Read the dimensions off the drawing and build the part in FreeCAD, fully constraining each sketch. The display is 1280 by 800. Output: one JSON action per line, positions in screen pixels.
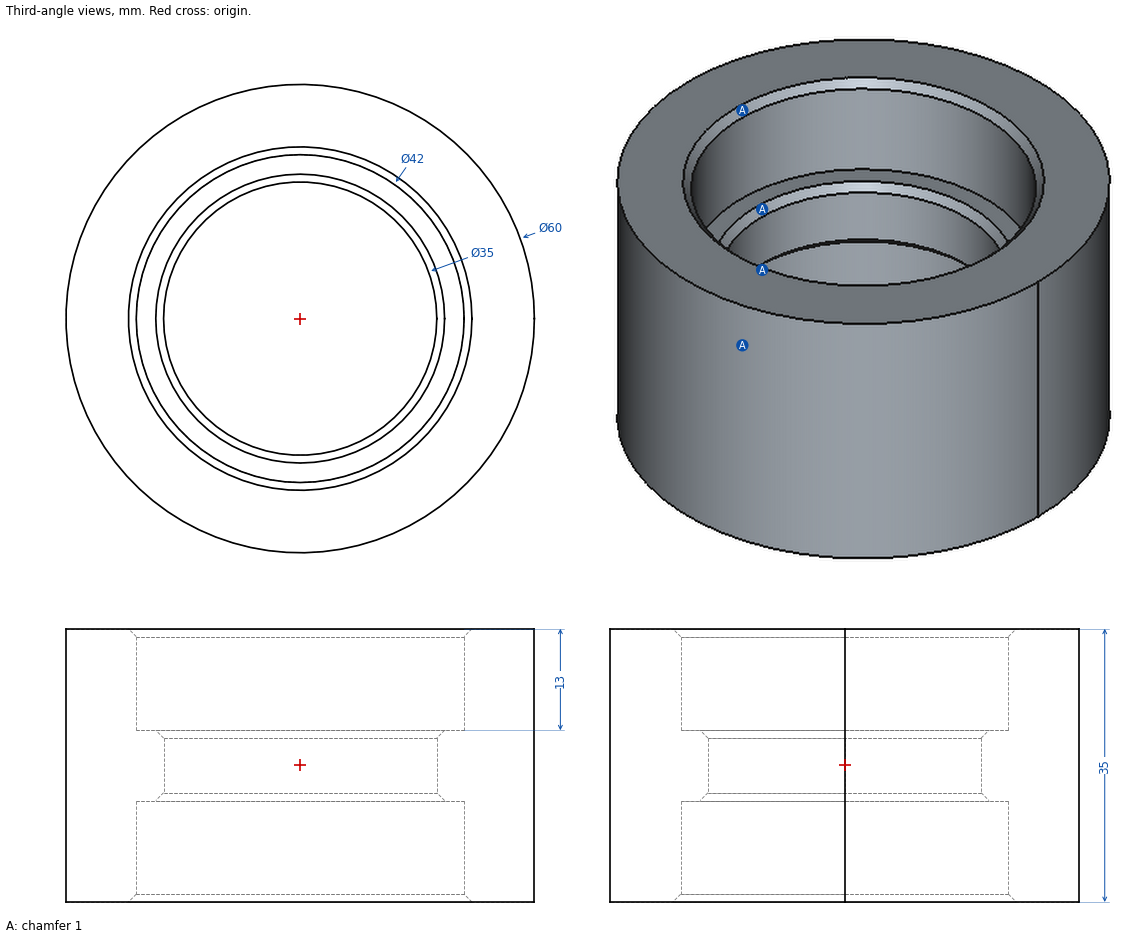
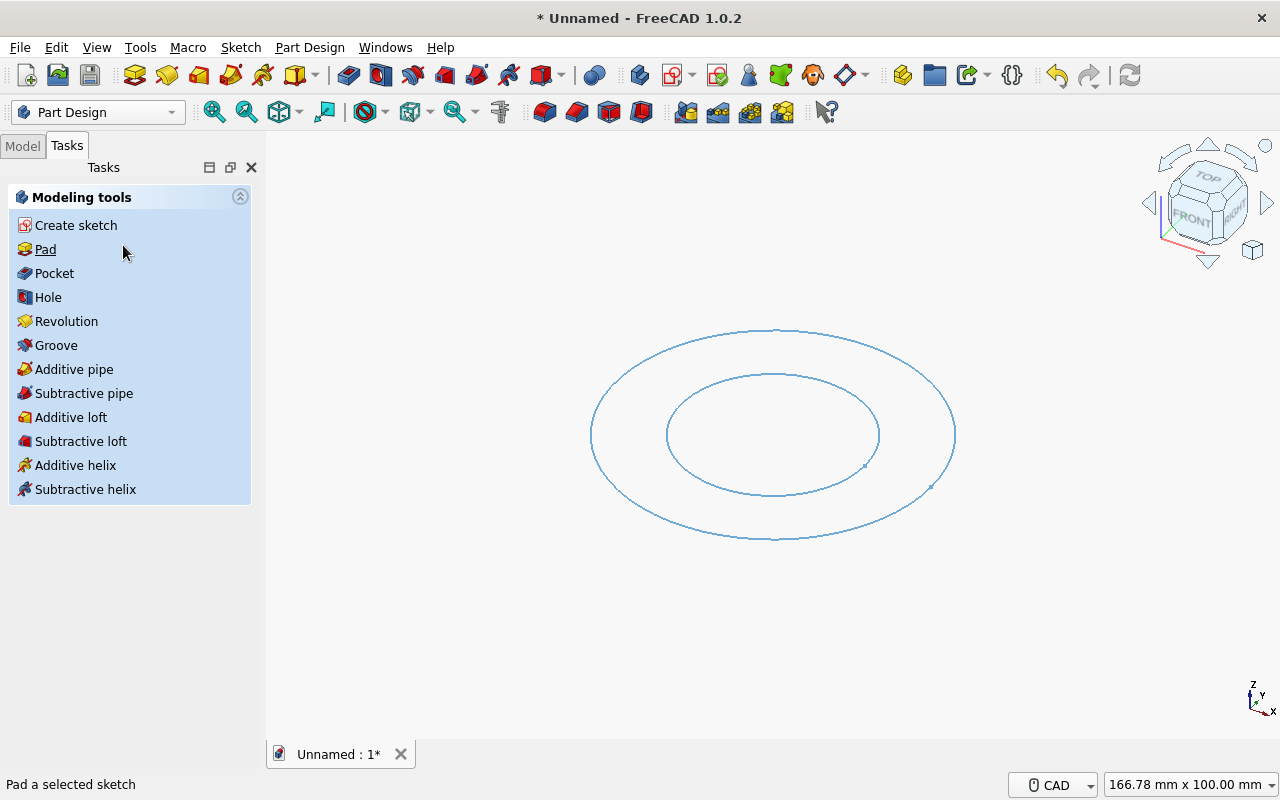
{"action": "left_click", "coordinate": [136, 76]}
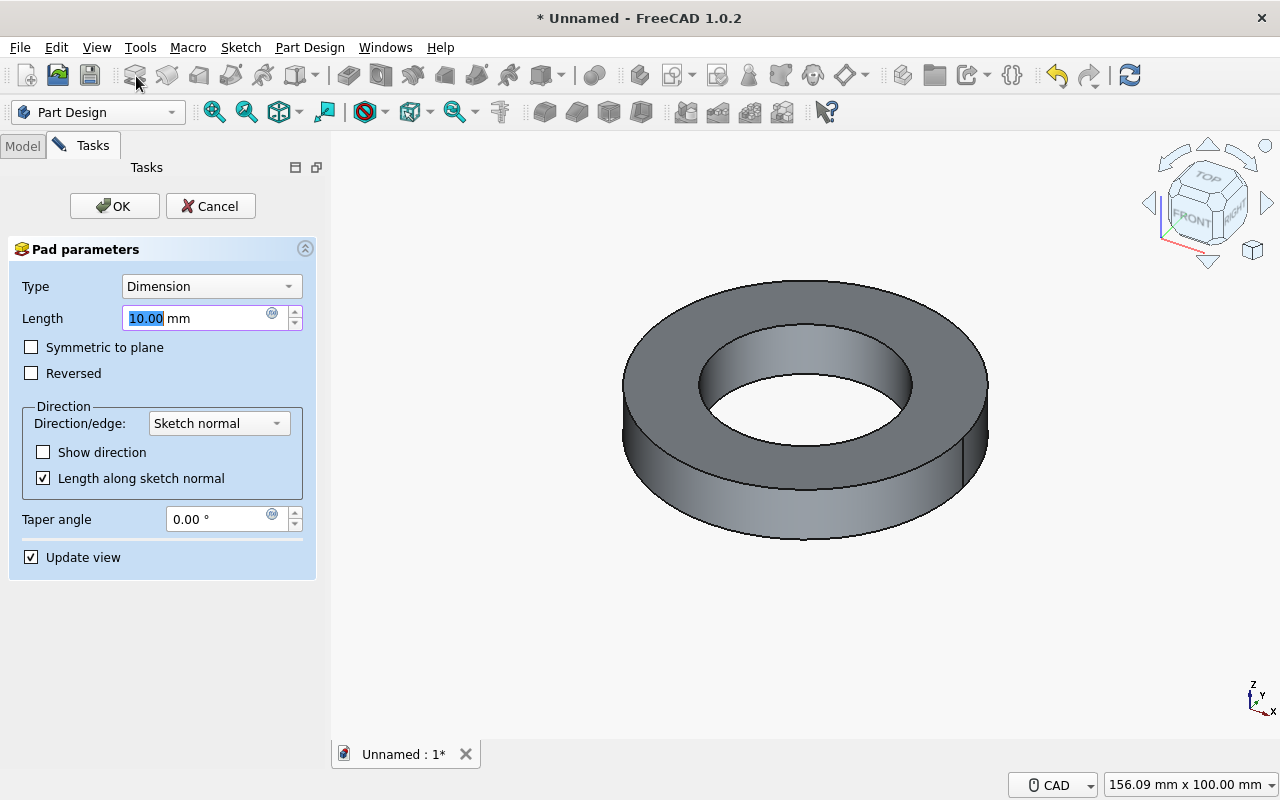
{"action": "type", "text": "35"}
{"action": "key", "text": "Tab"}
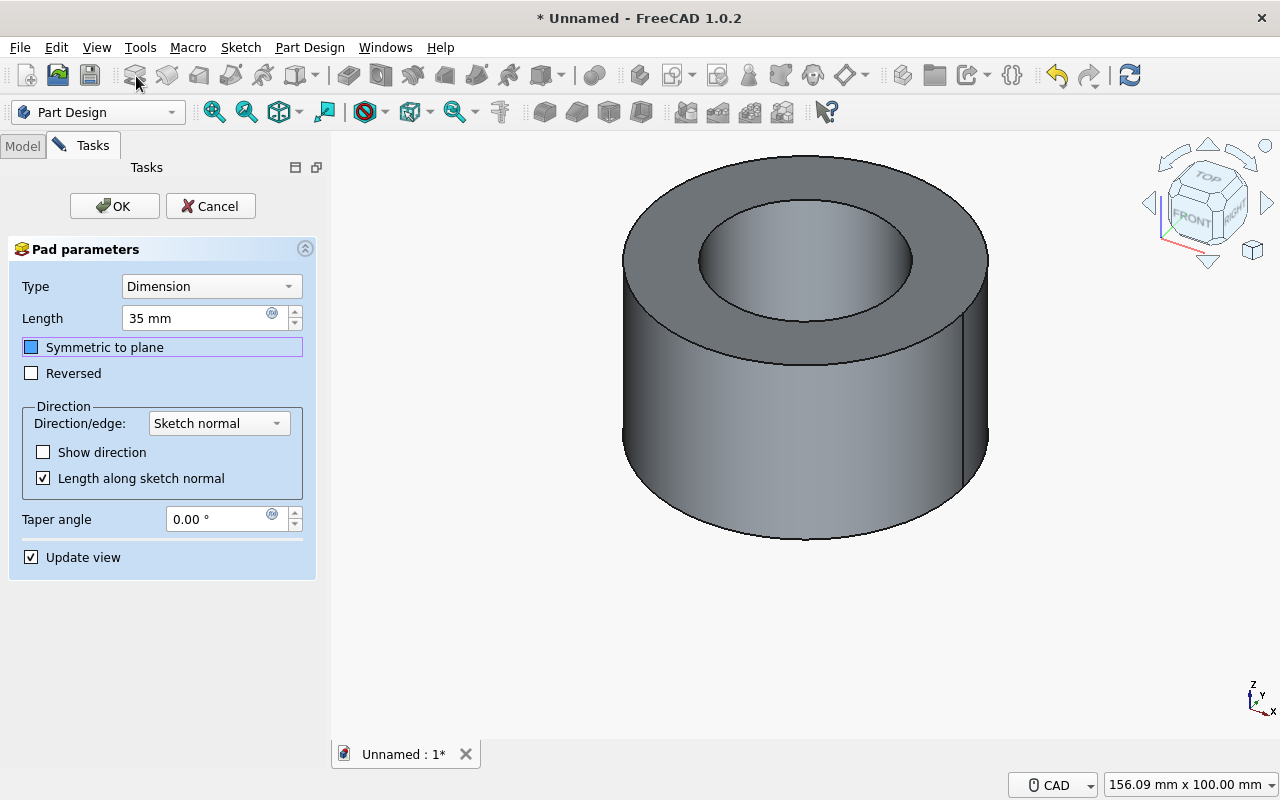
{"action": "left_click", "coordinate": [30, 347]}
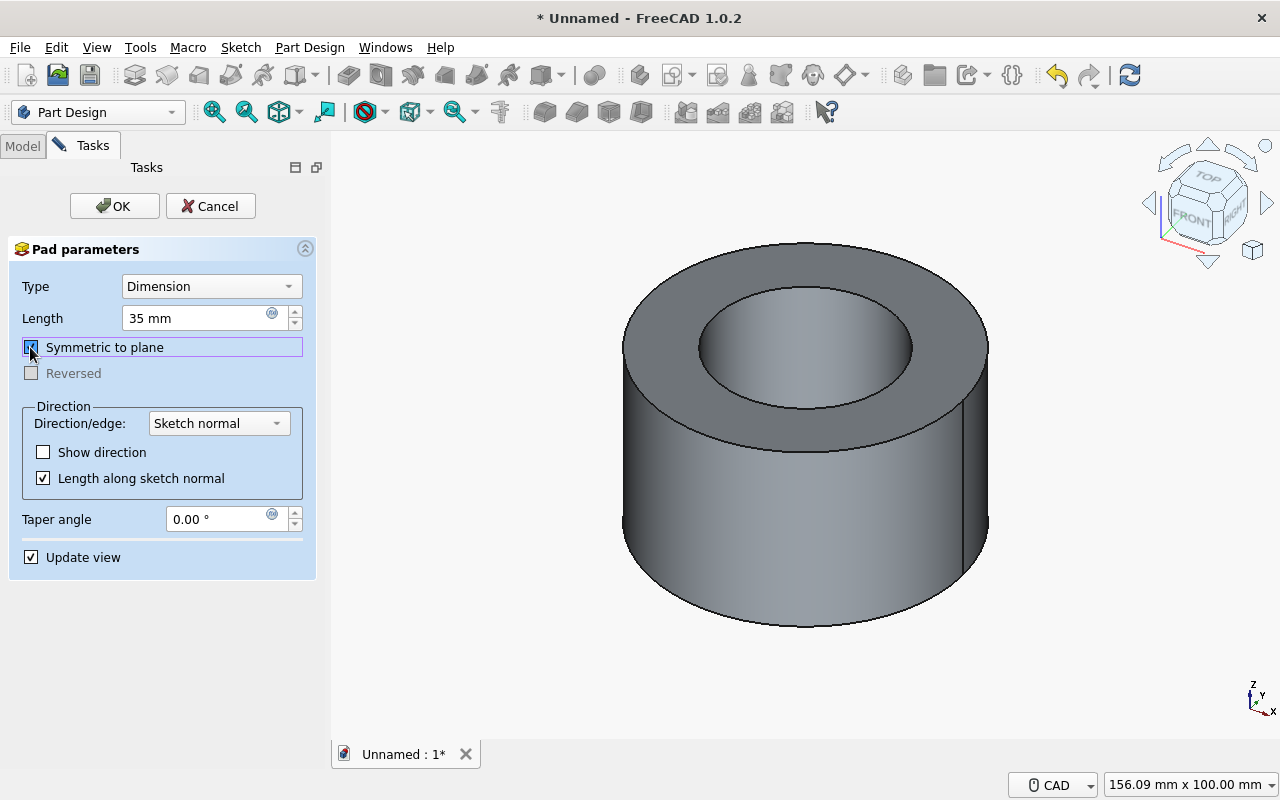
{"action": "left_click", "coordinate": [115, 206]}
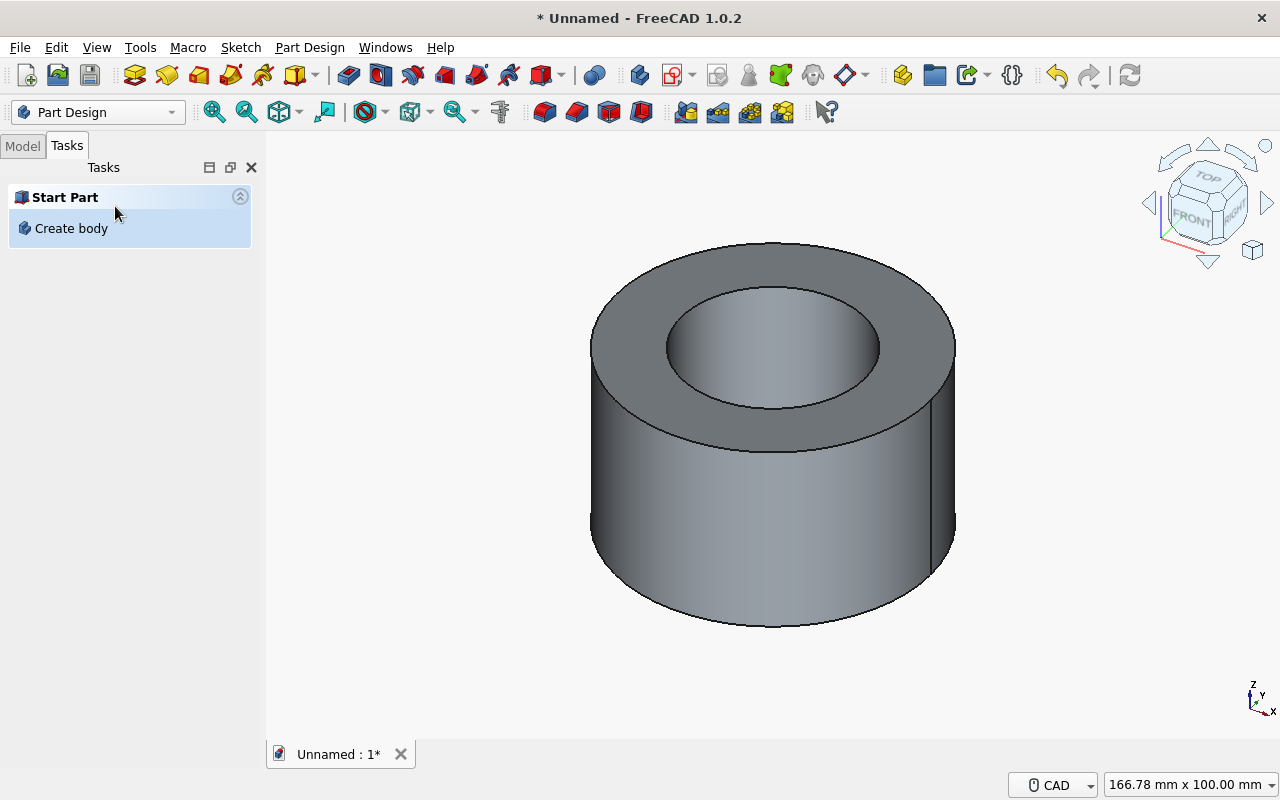
{"action": "left_click", "coordinate": [631, 369]}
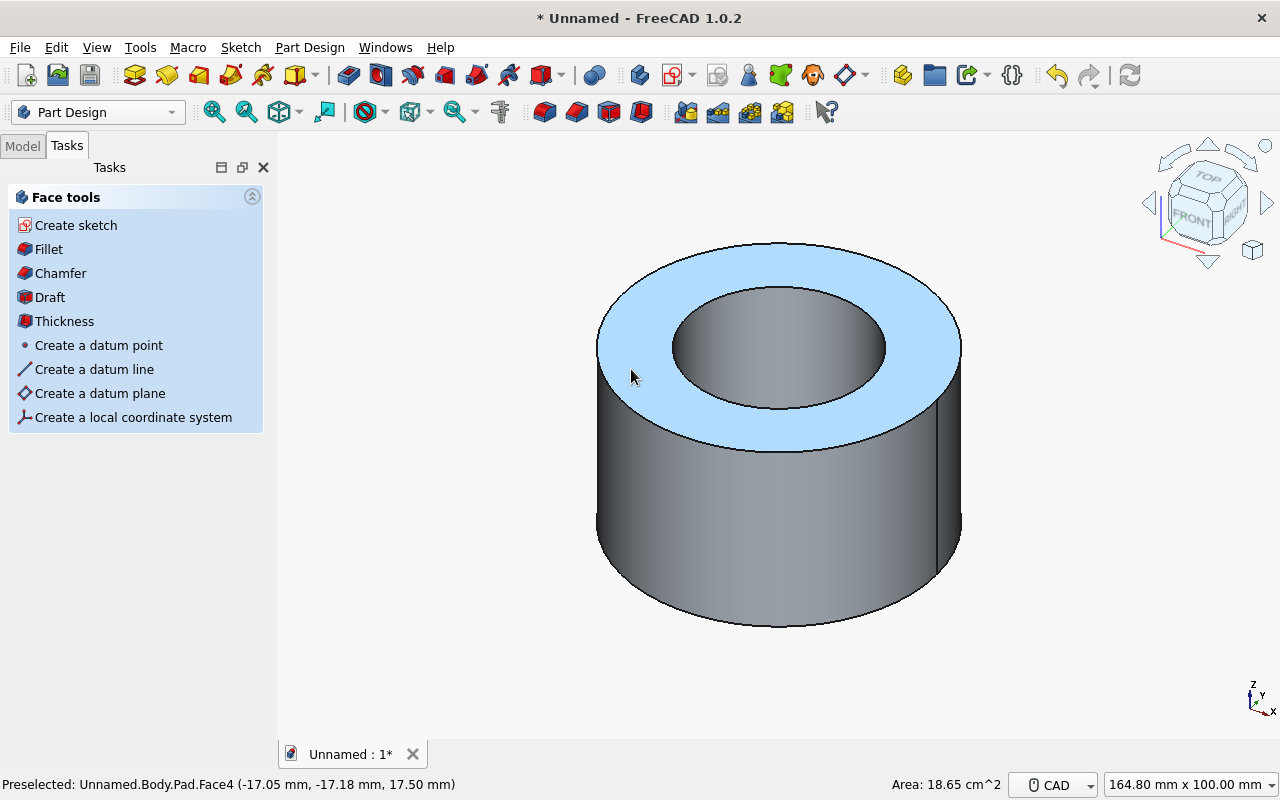
{"action": "left_click", "coordinate": [672, 76]}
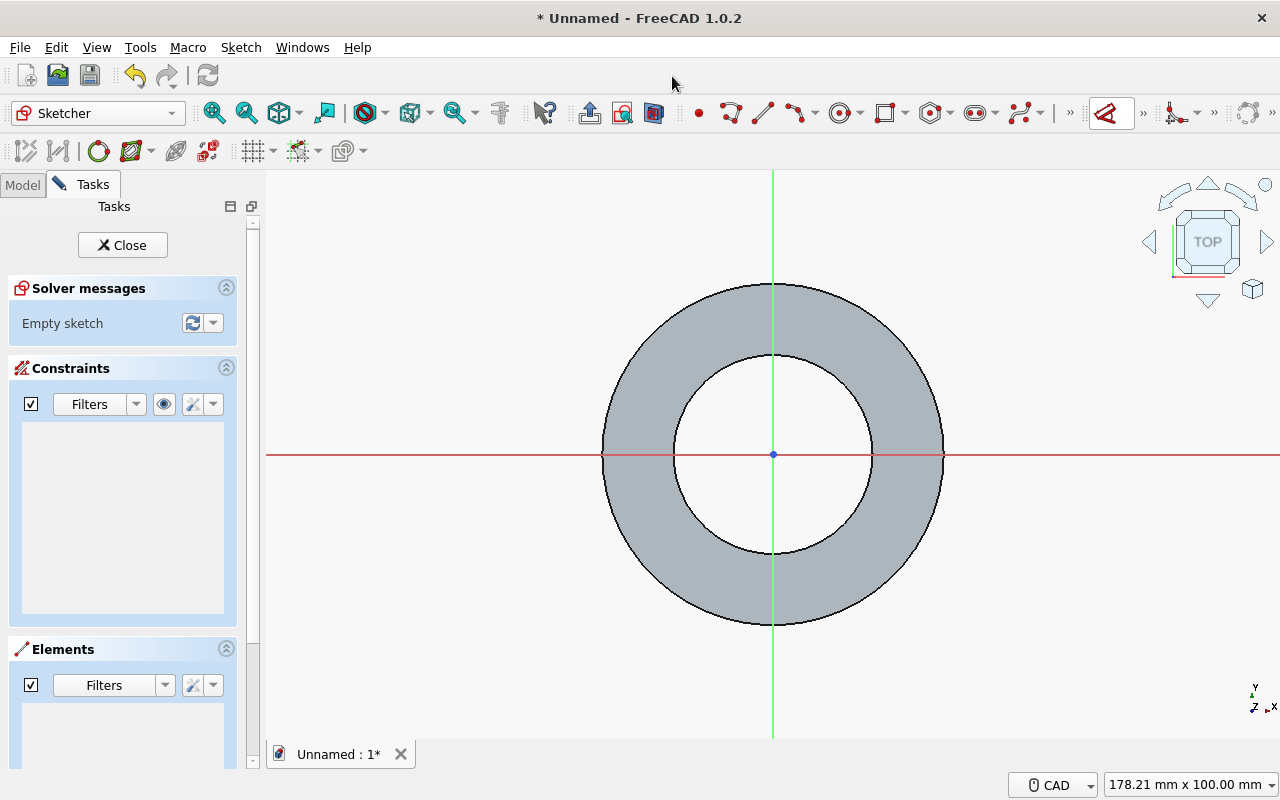
{"action": "scroll", "coordinate": [912, 455], "scroll_direction": "up", "scroll_amount": 2}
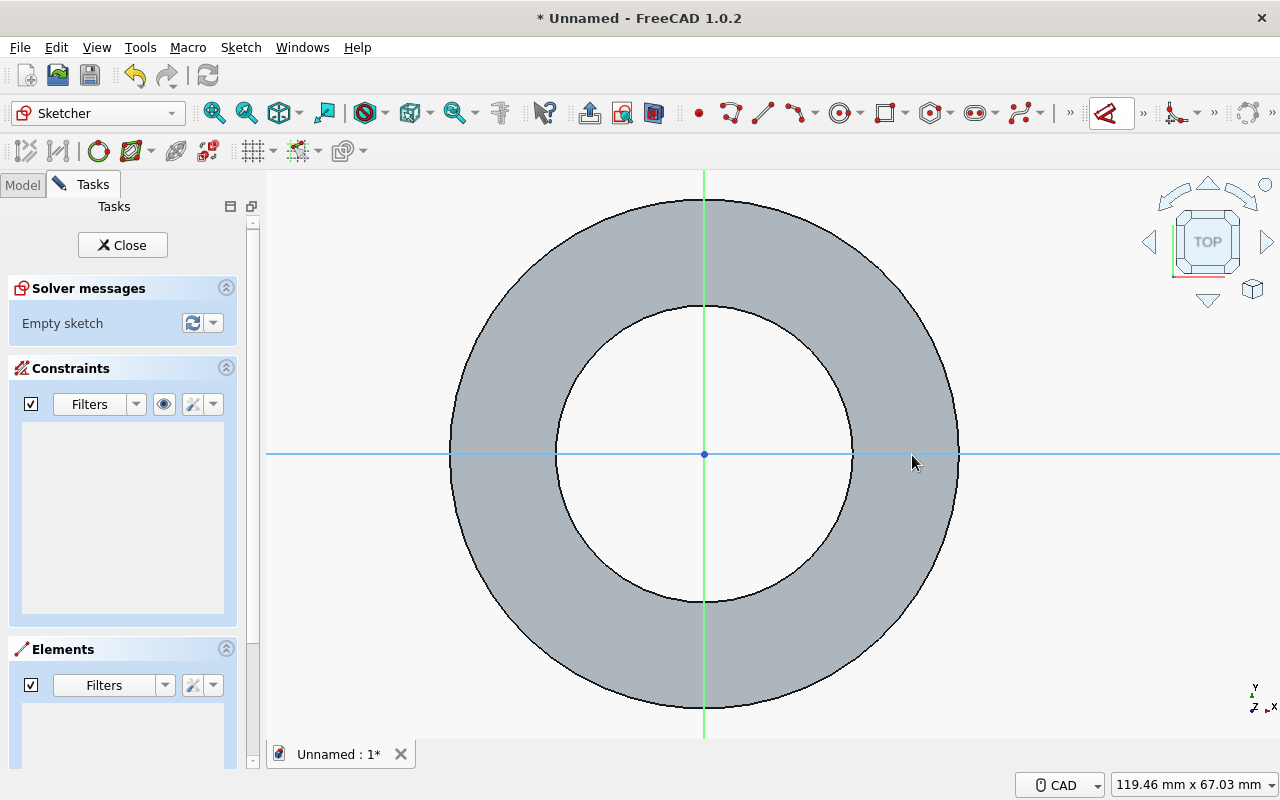
{"action": "left_click", "coordinate": [840, 114]}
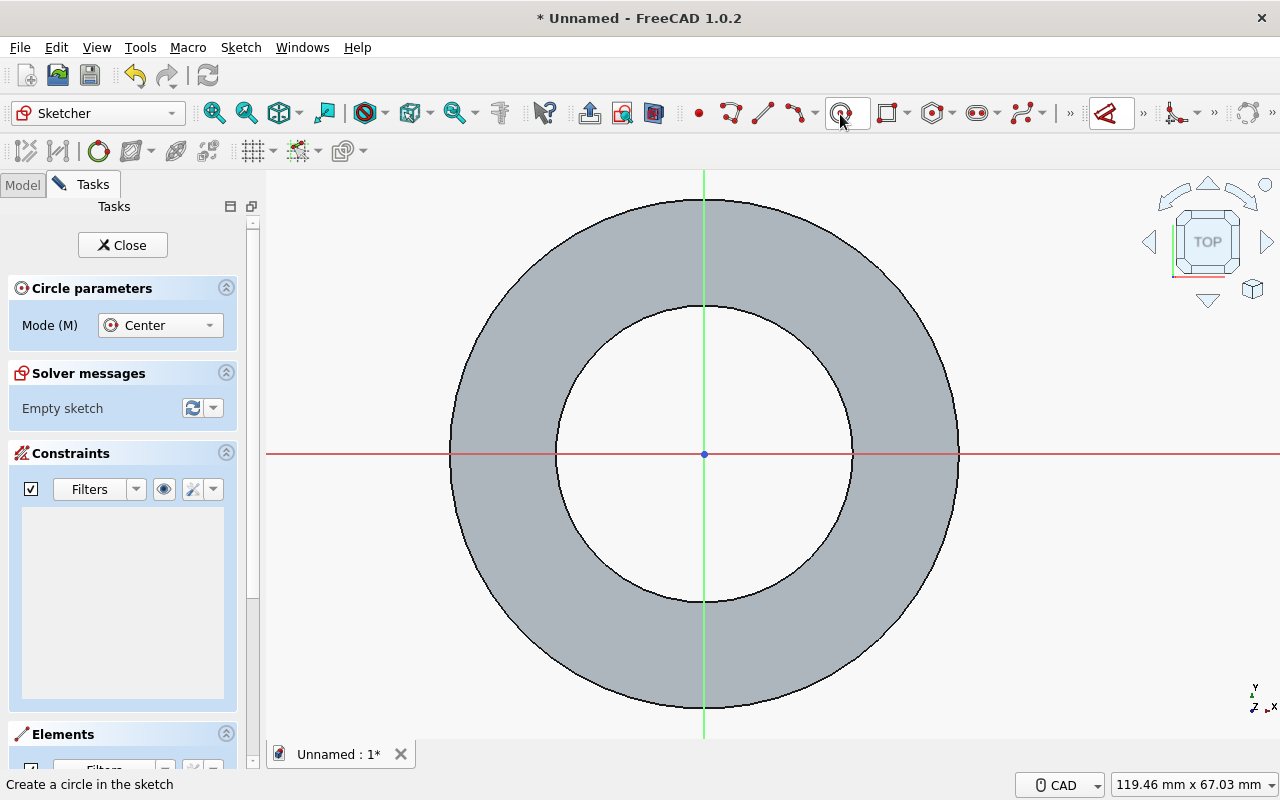
{"action": "left_click", "coordinate": [704, 454]}
{"action": "mouse_move", "coordinate": [830, 328]}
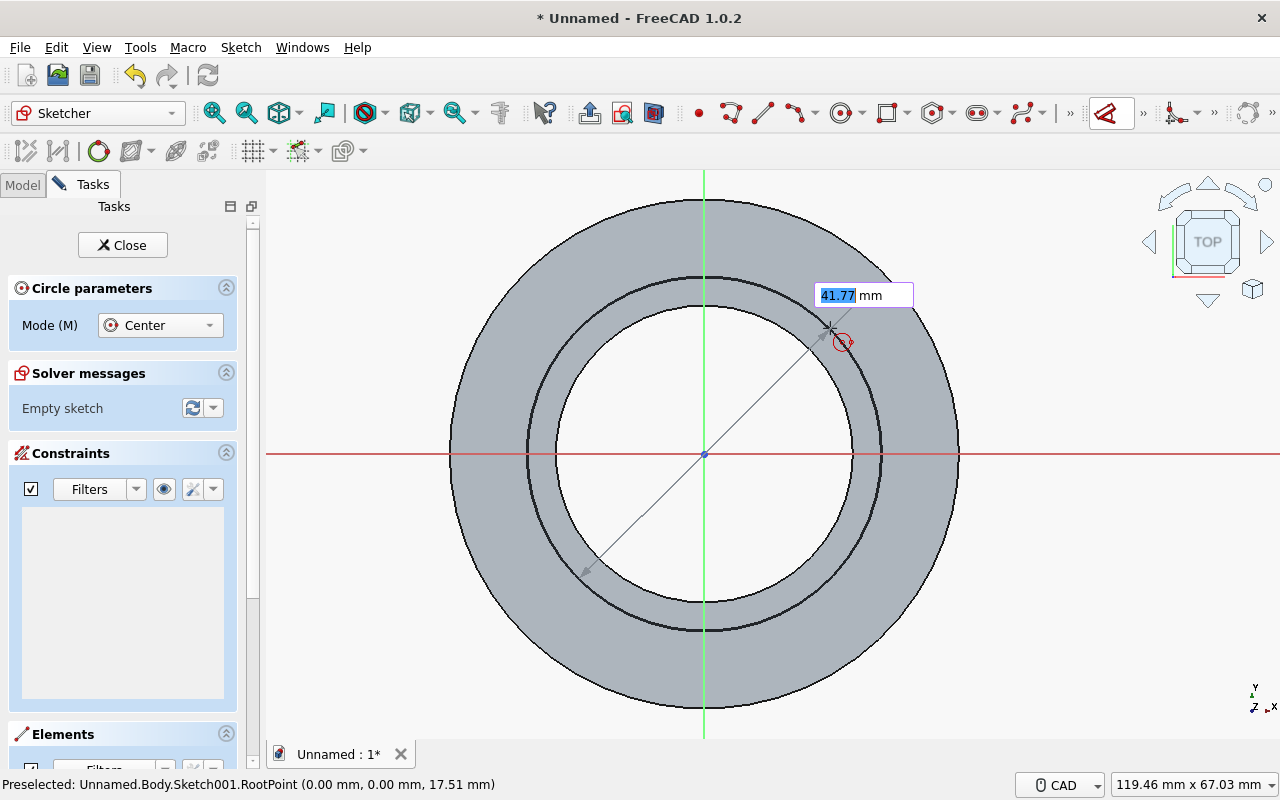
{"action": "type", "text": "42"}
{"action": "key", "text": "Return"}
{"action": "key", "text": "Escape"}